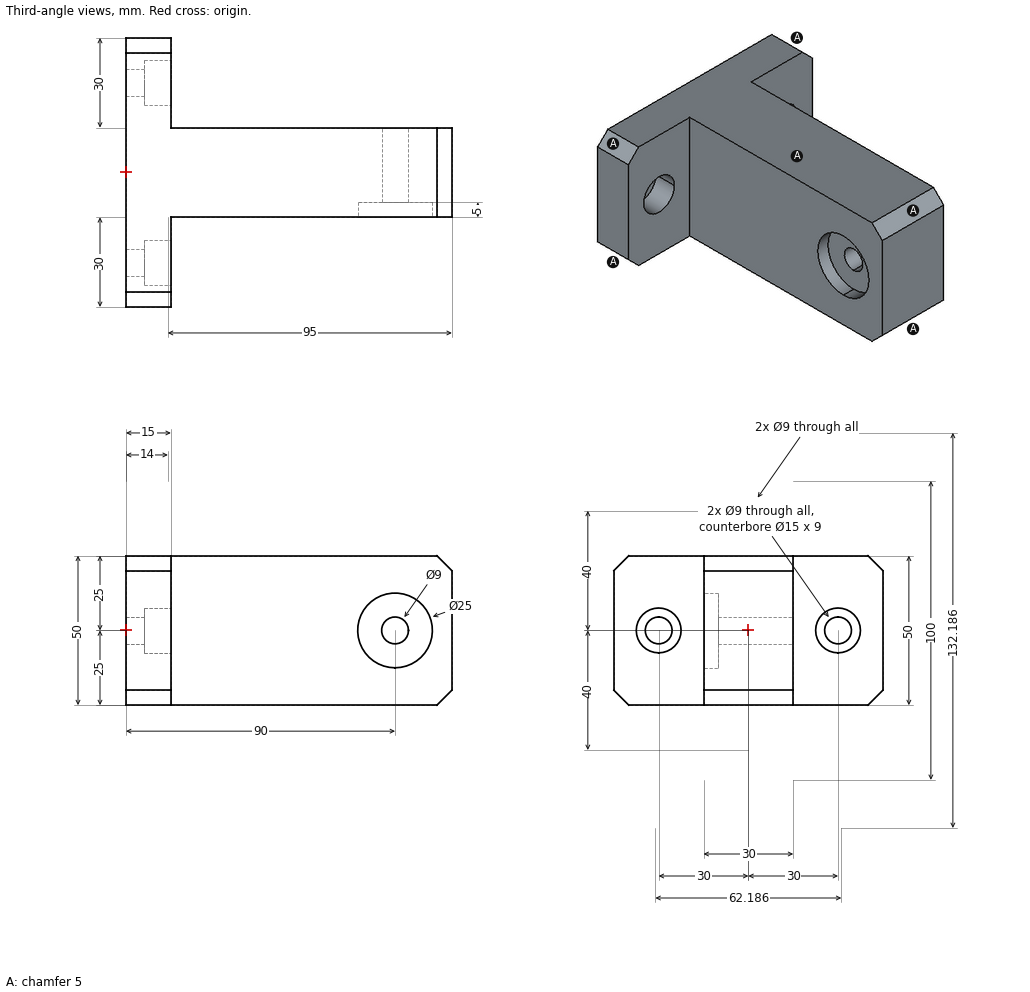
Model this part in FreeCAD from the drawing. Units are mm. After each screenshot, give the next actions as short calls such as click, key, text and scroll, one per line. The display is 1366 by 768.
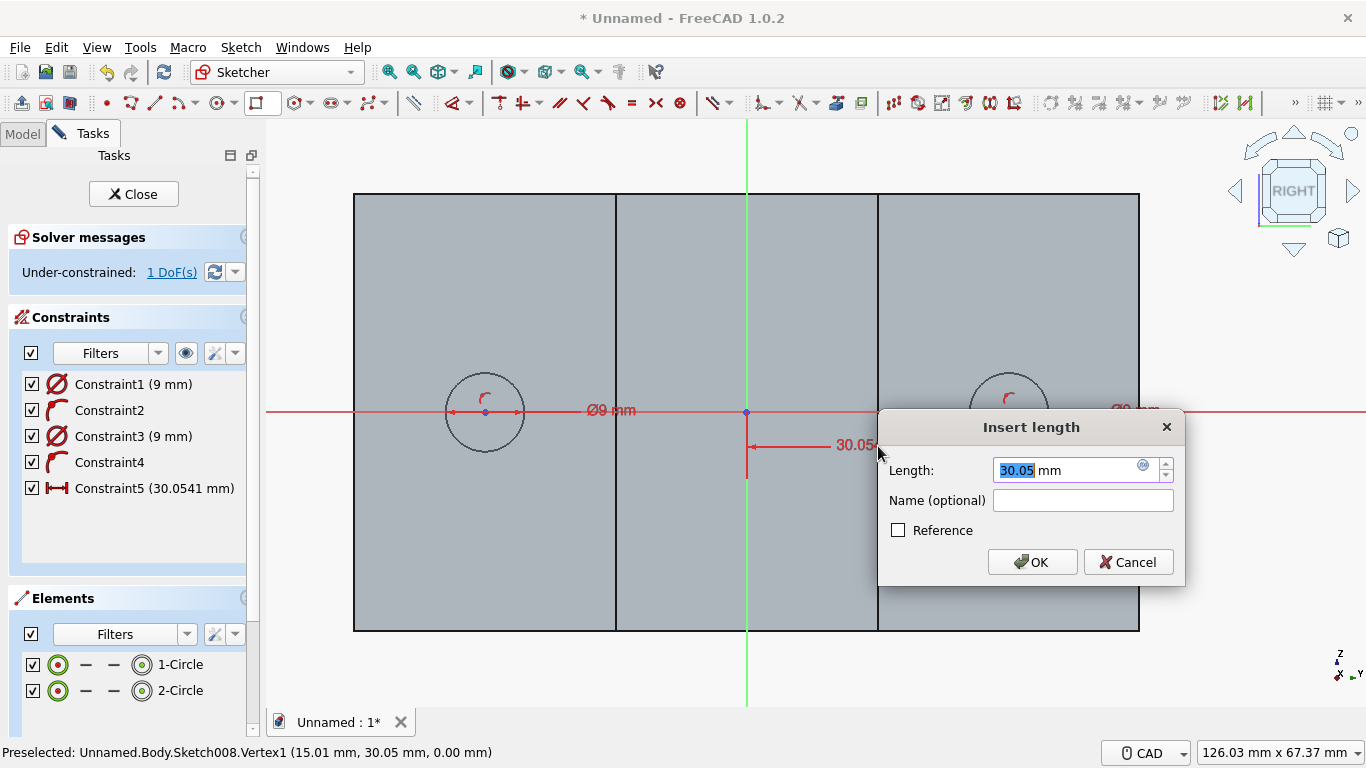
text(30)
key(Return)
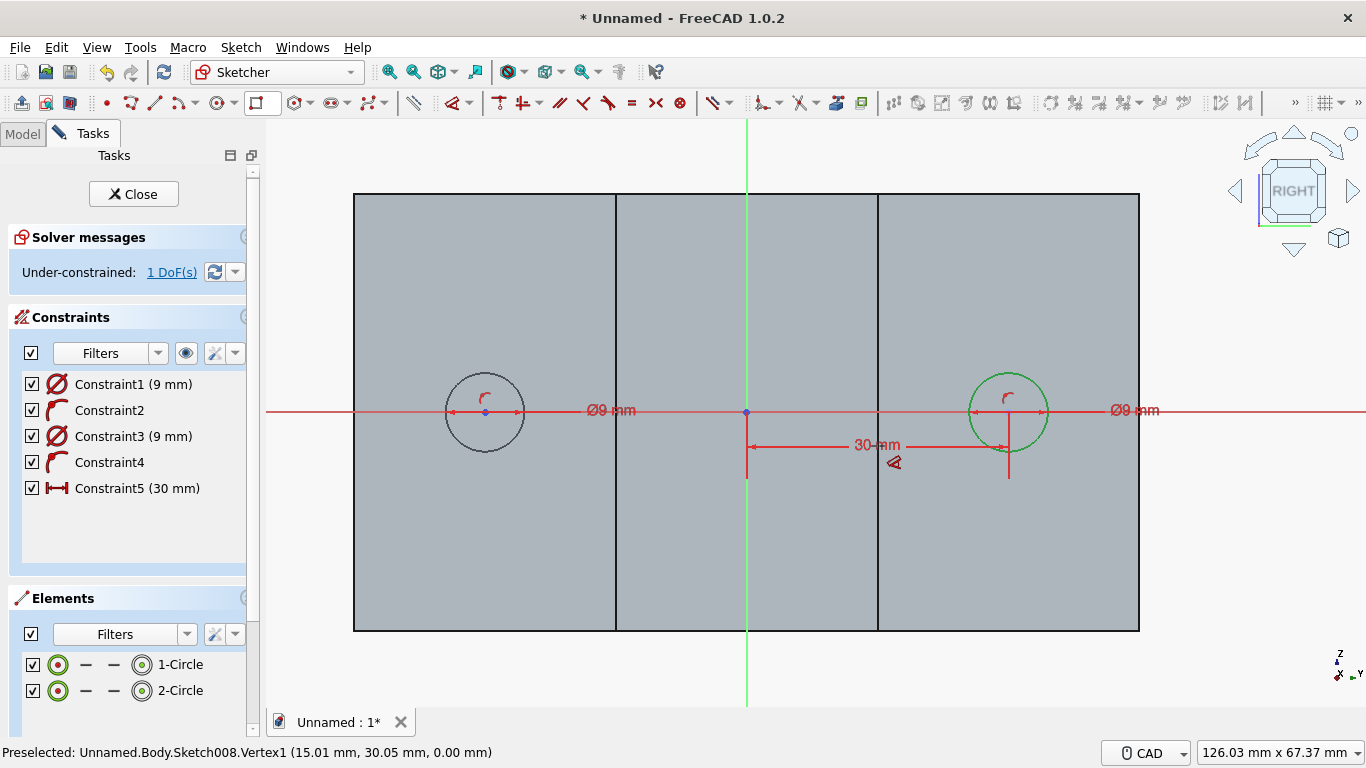
click(485, 412)
click(616, 446)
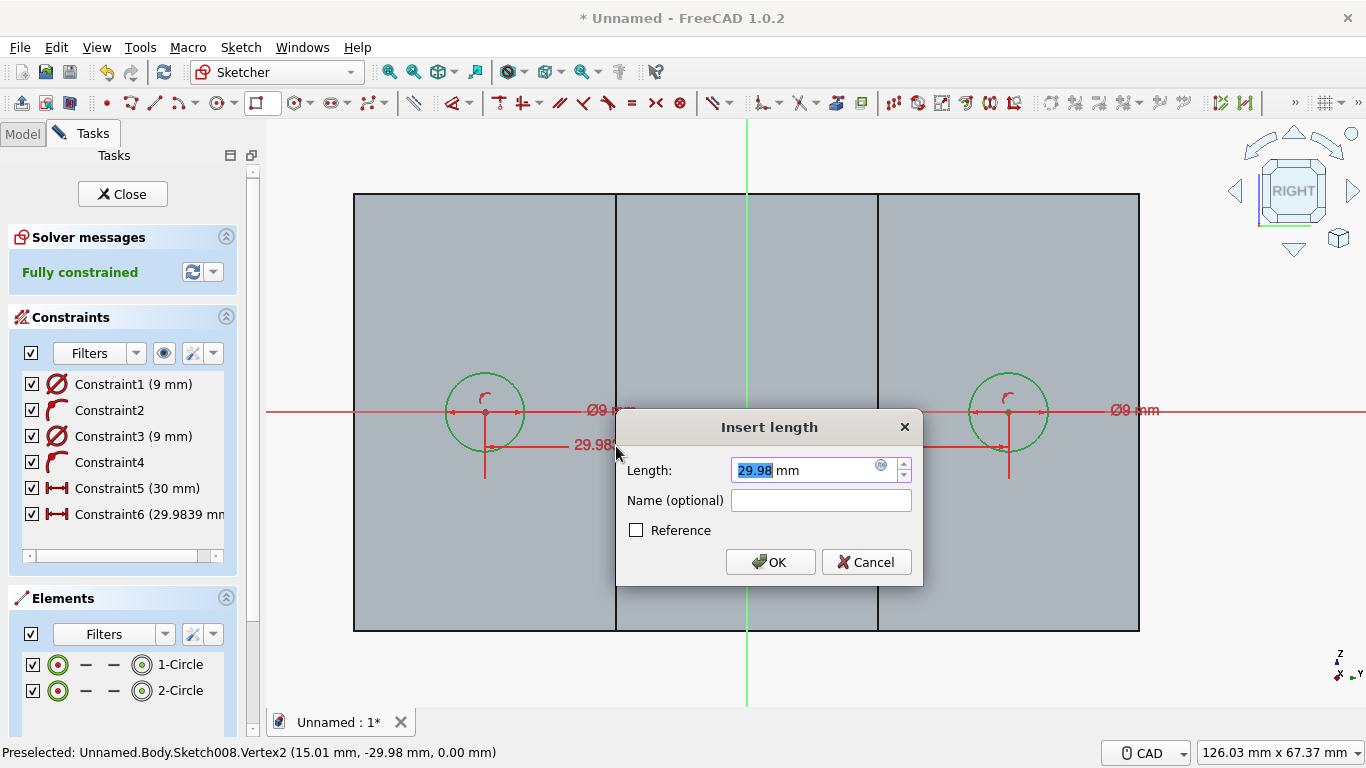
text(30)
key(Return)
key(Escape)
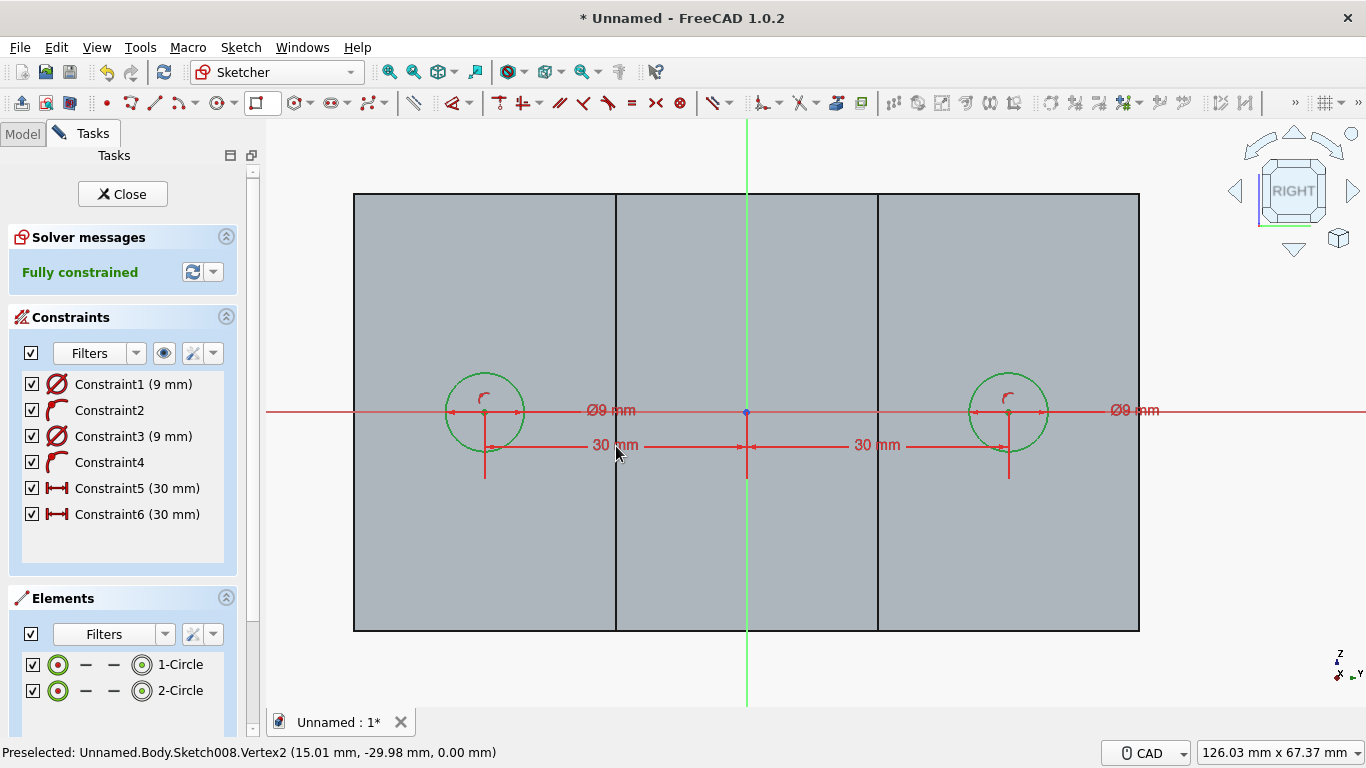
click(123, 194)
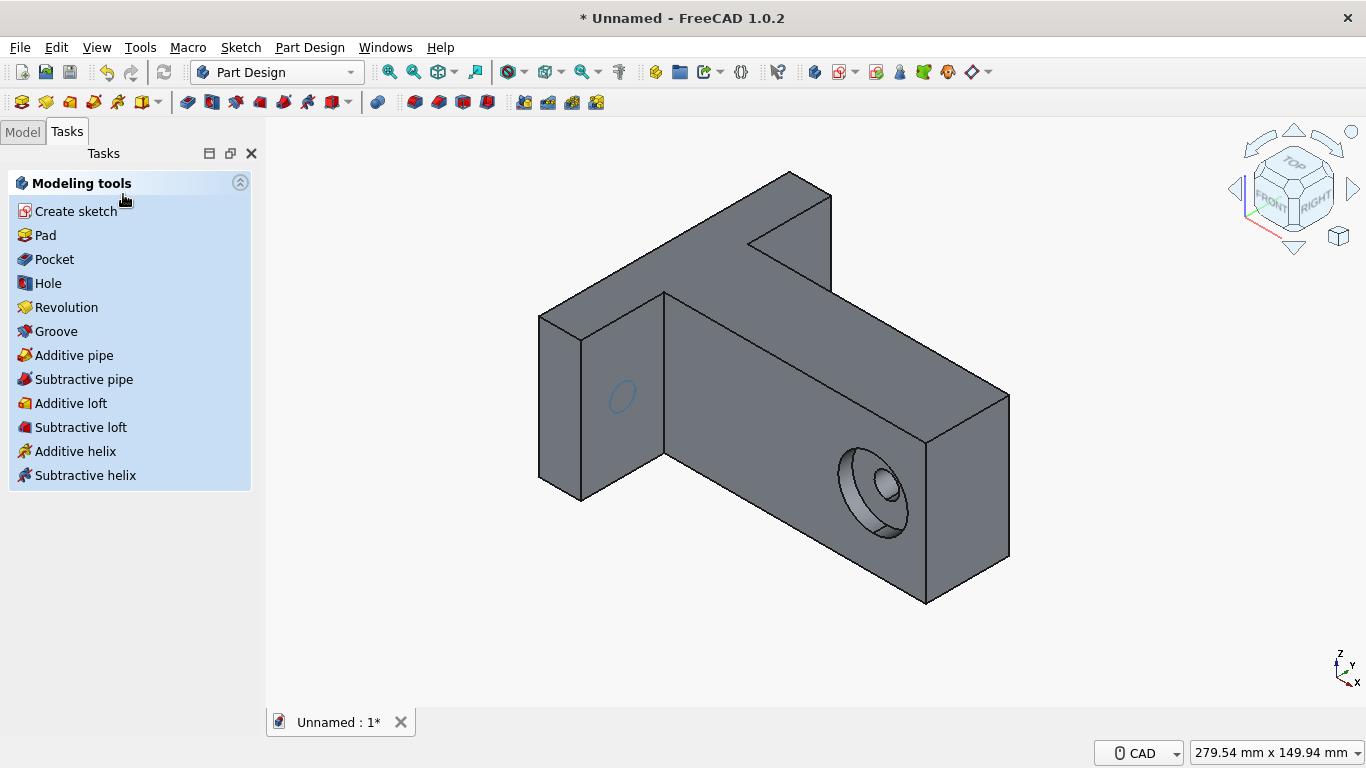
click(212, 102)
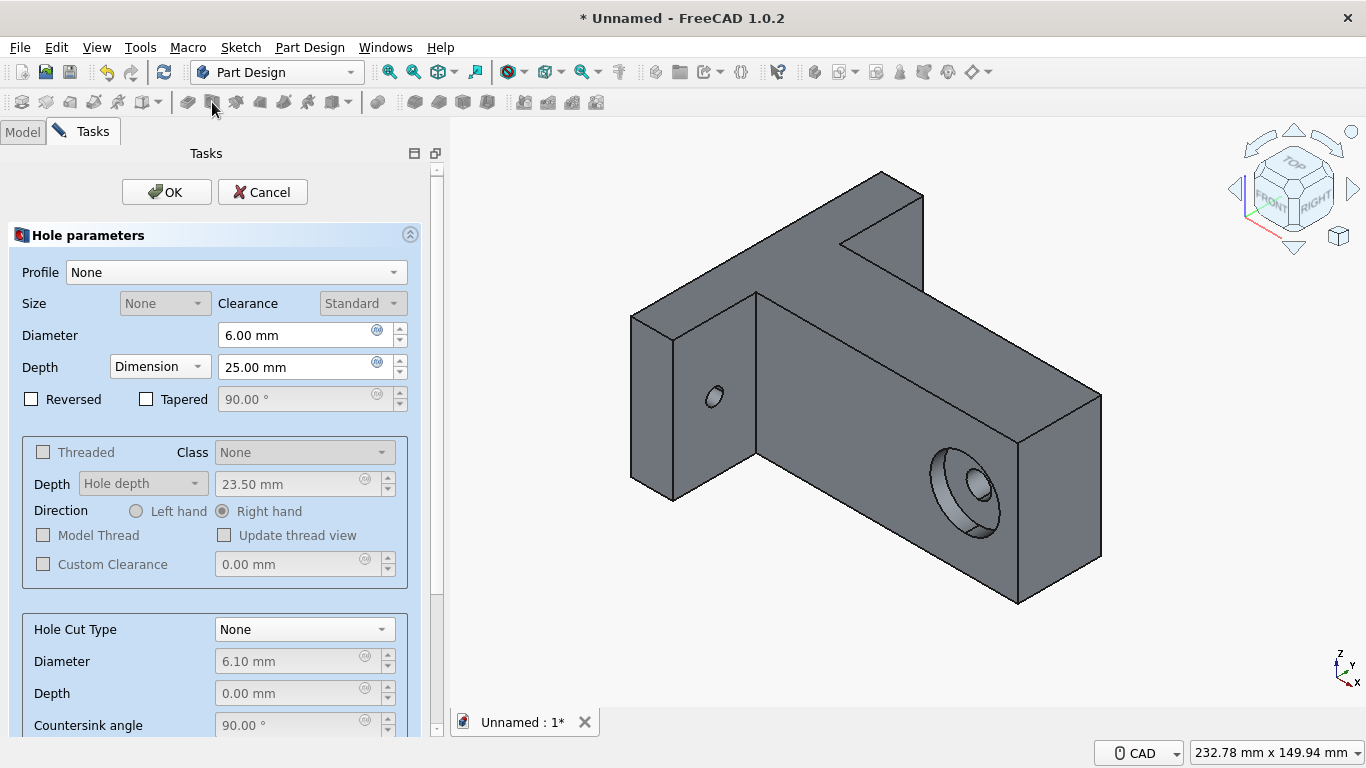
triple_click(305, 335)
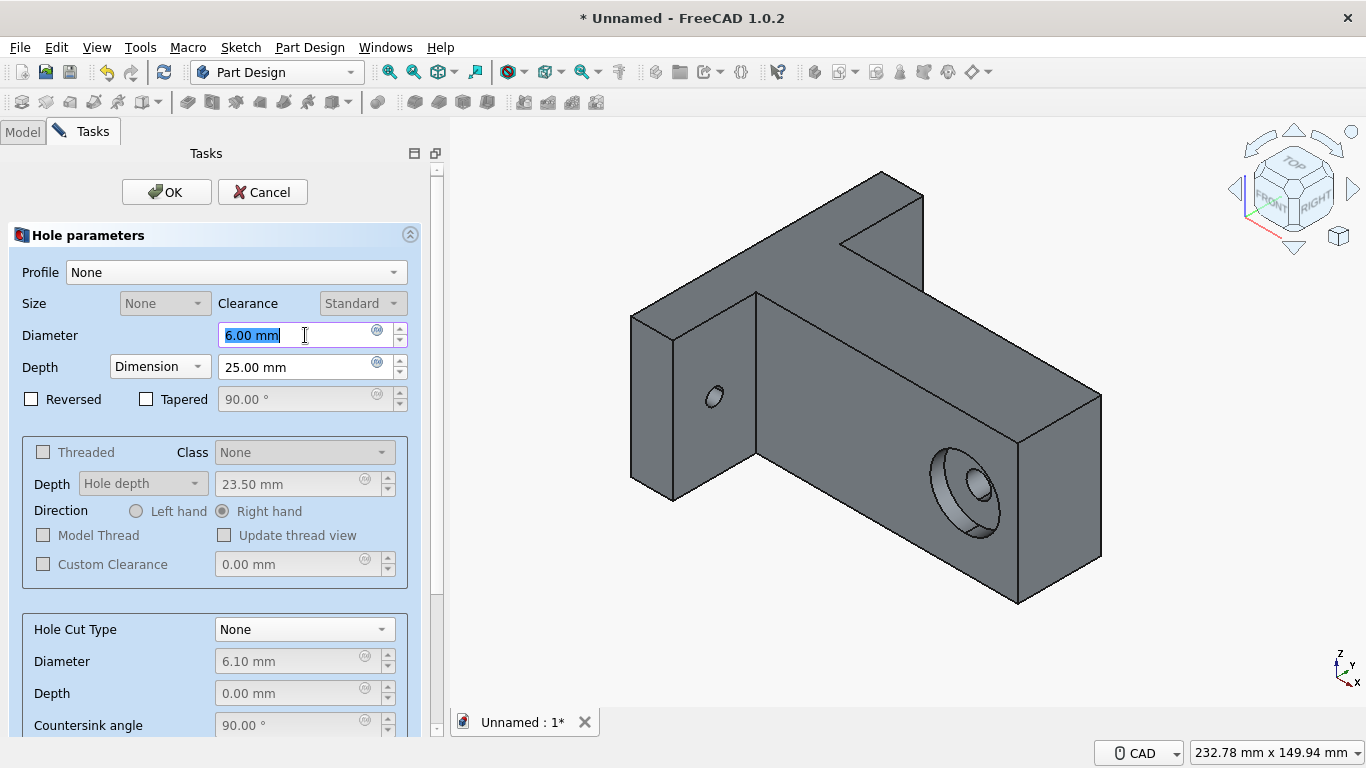
text(9)
key(Tab)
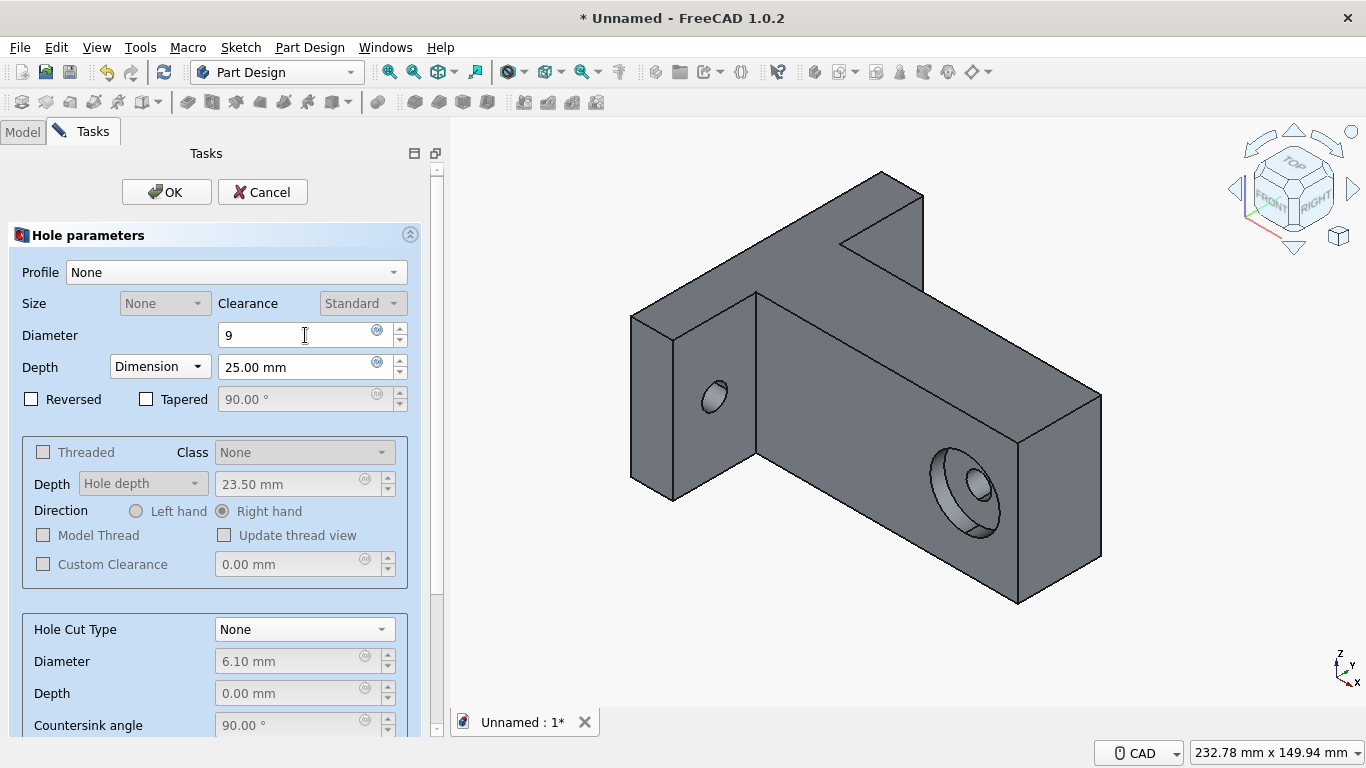
click(161, 366)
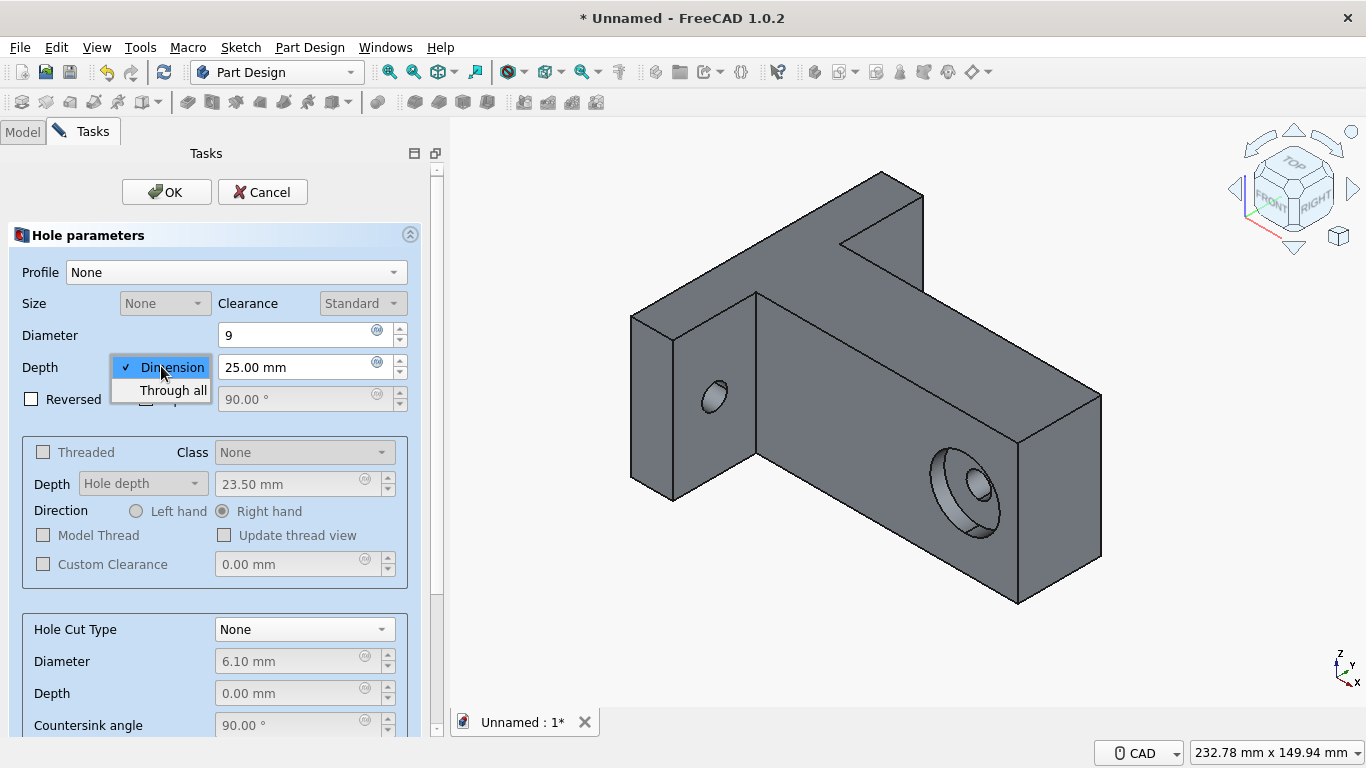
click(160, 390)